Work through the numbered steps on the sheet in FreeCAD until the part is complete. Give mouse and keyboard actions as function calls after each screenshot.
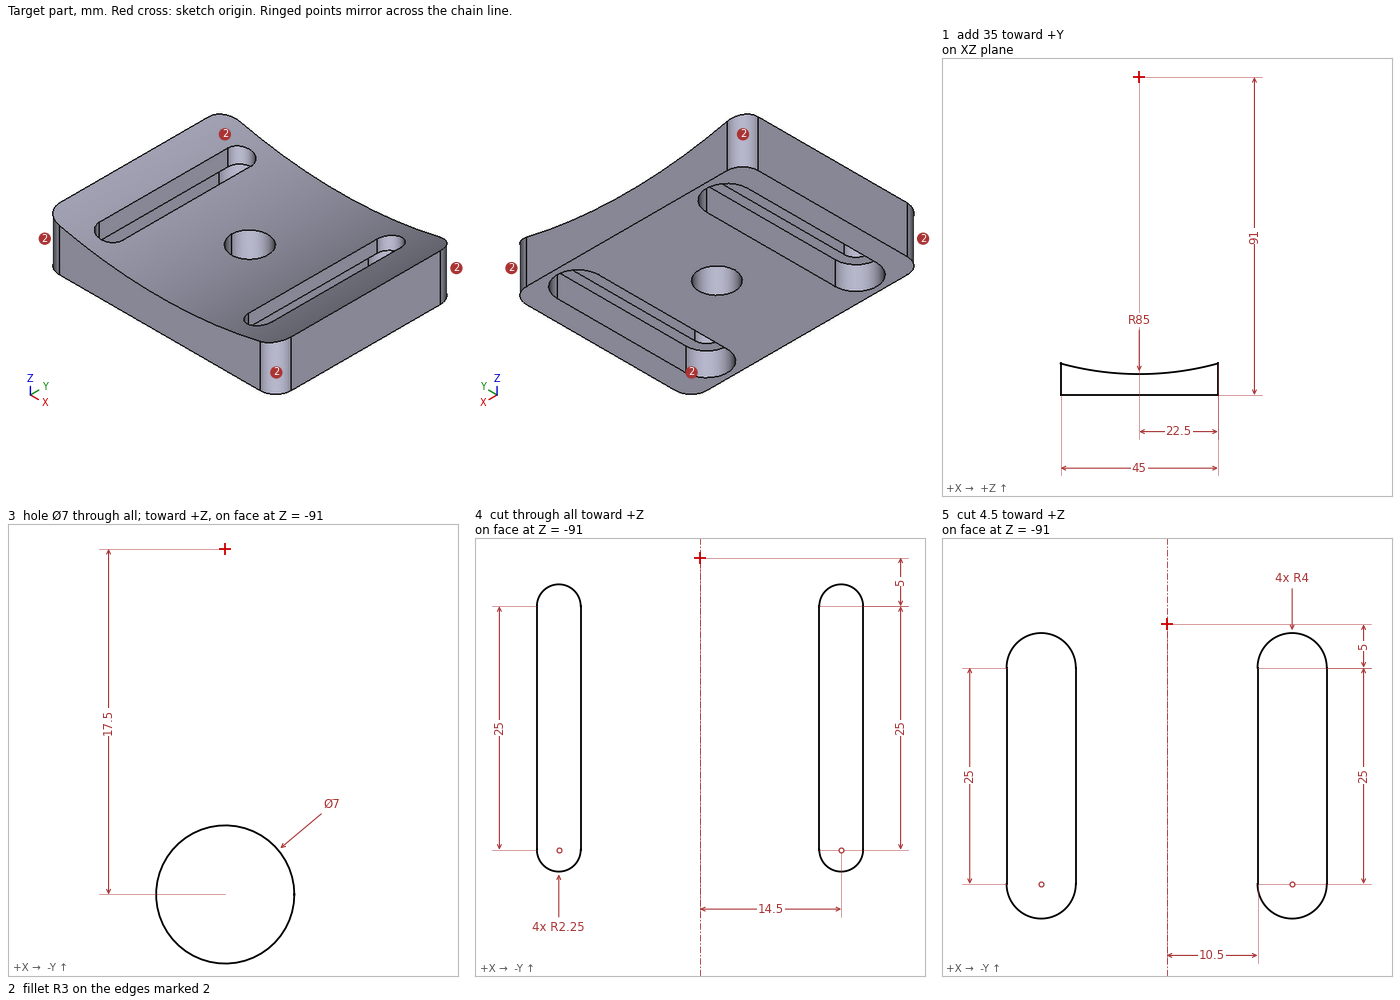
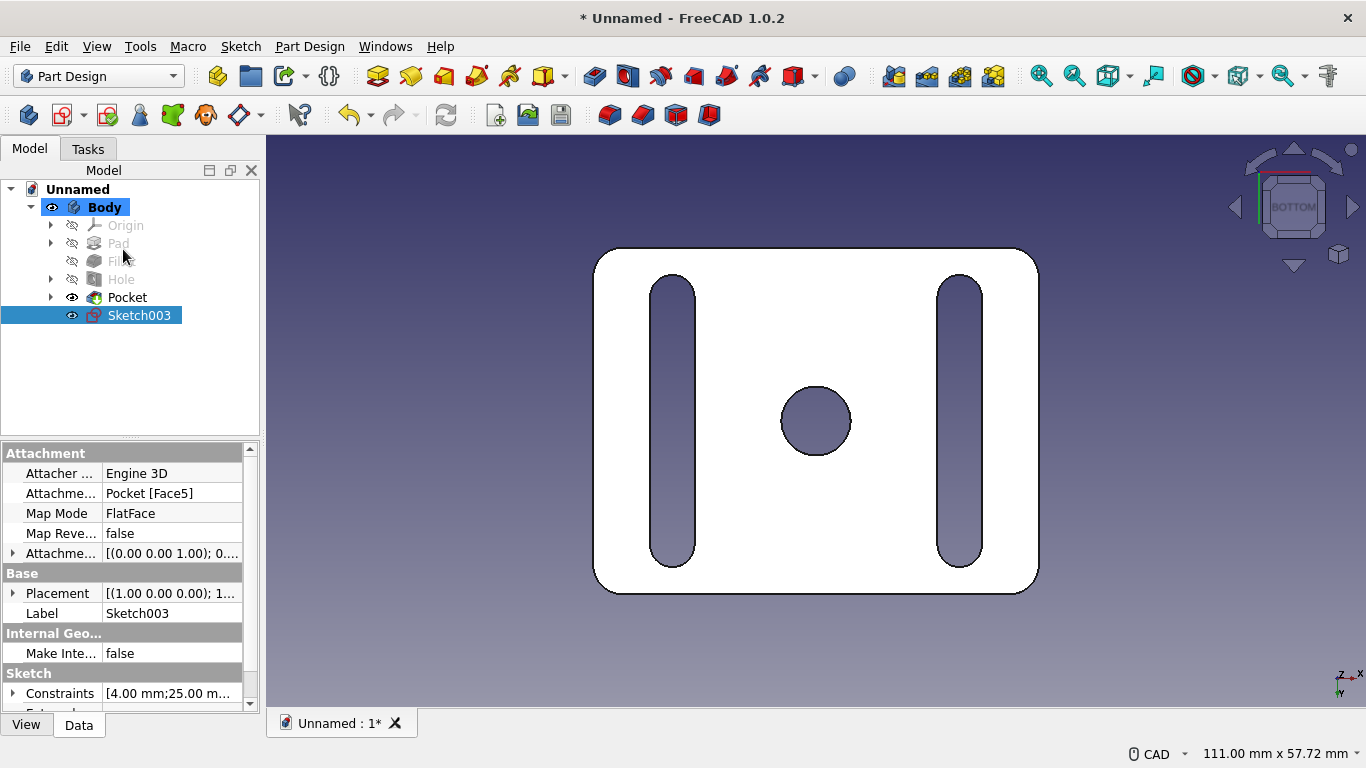
click(595, 76)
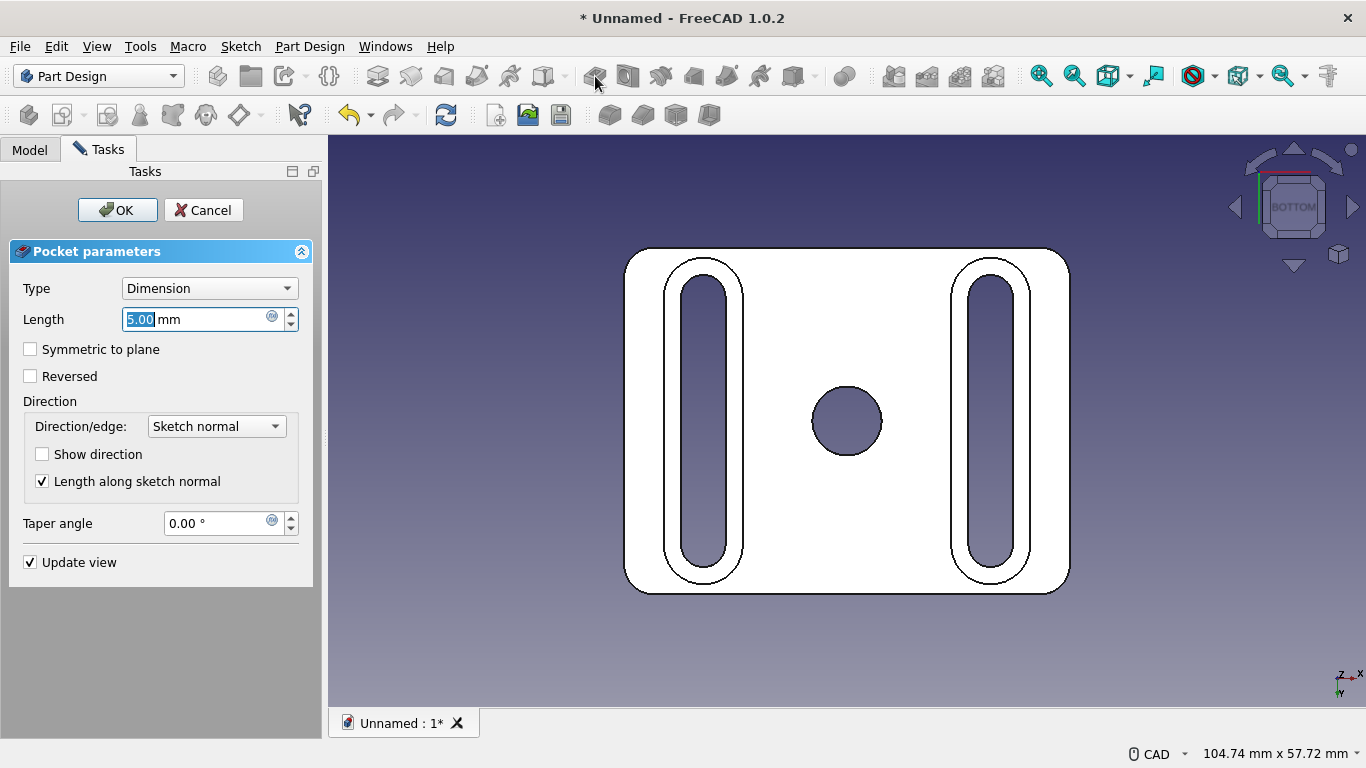
text(4.5)
key(Tab)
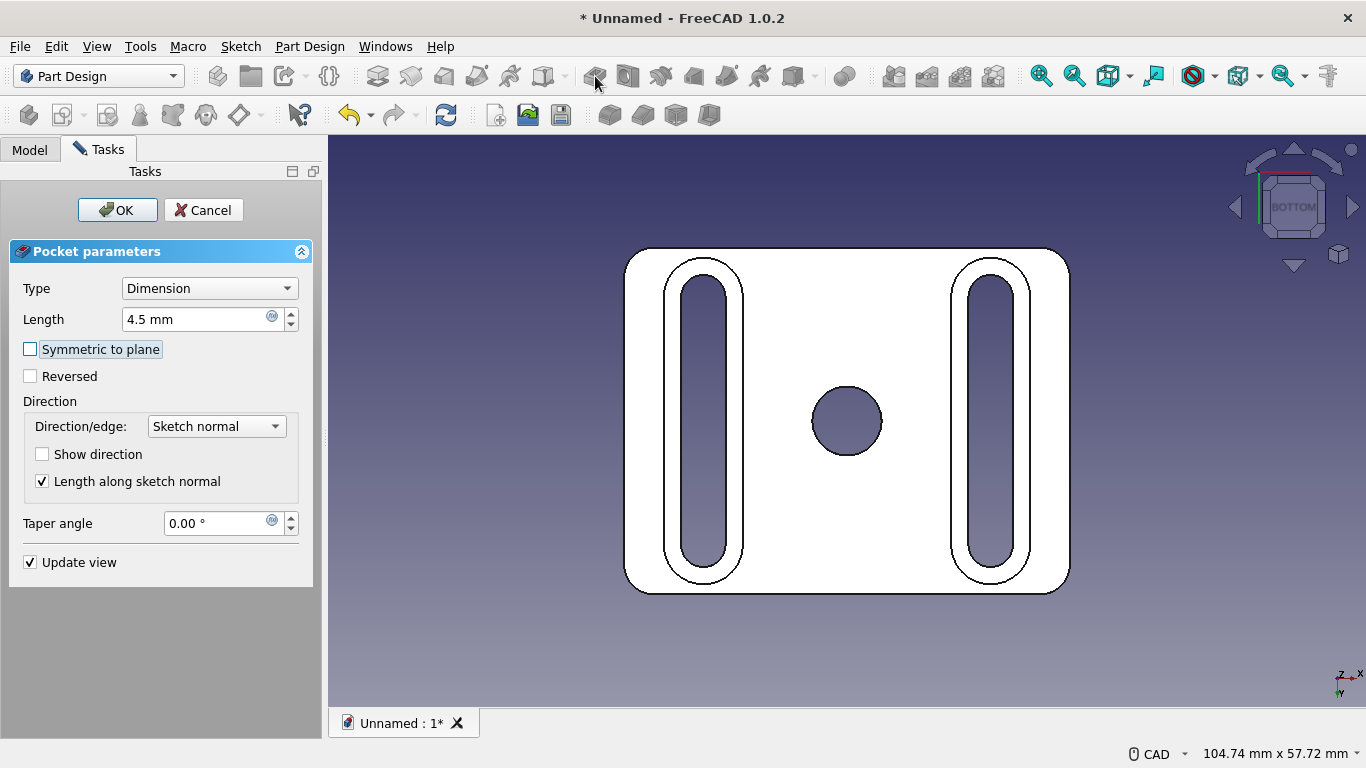
click(118, 210)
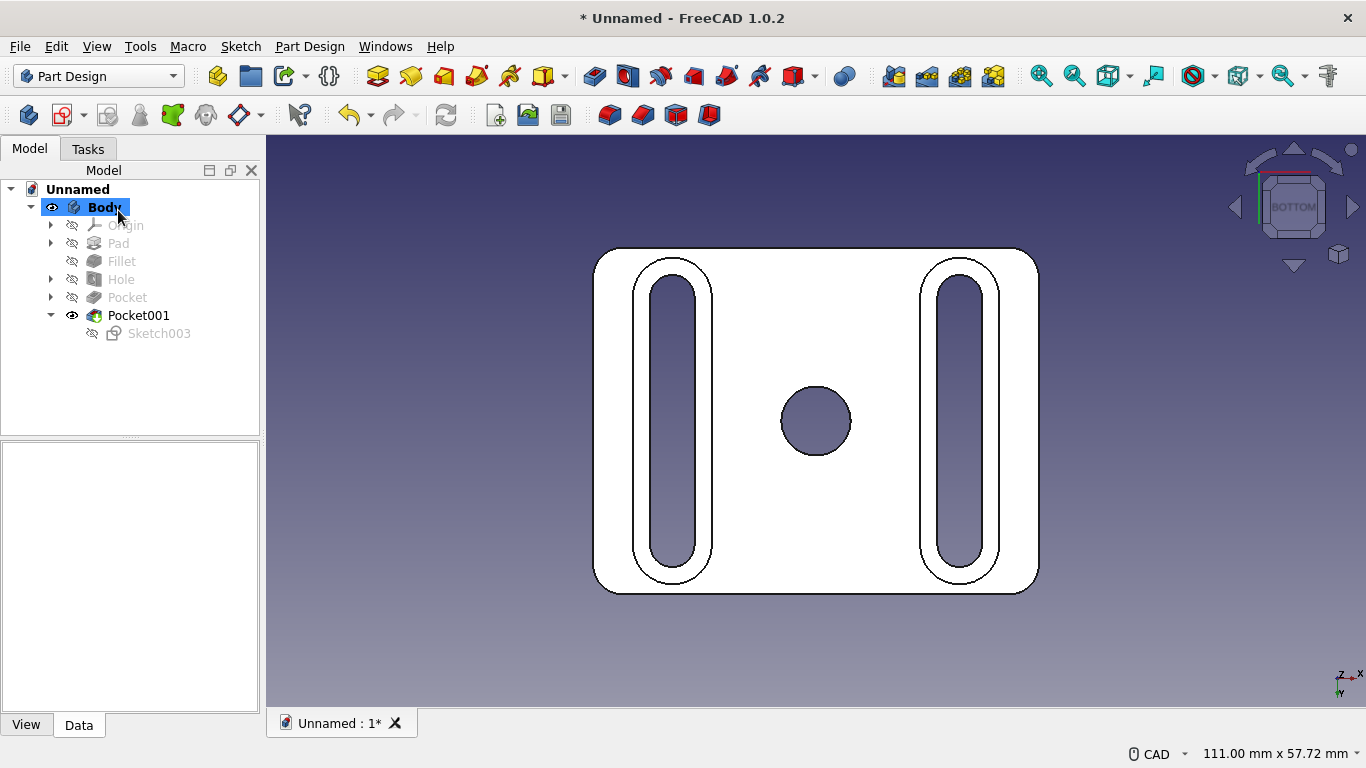
key(0)